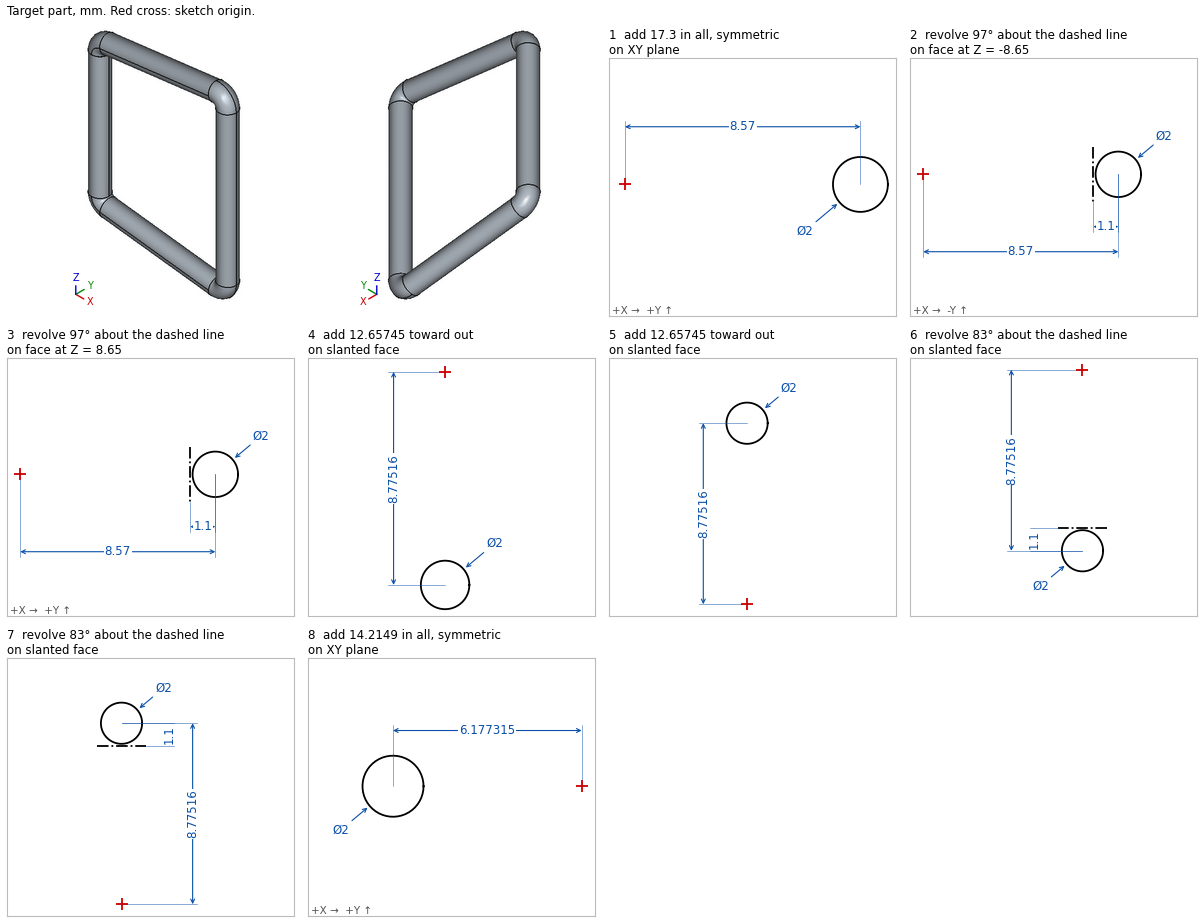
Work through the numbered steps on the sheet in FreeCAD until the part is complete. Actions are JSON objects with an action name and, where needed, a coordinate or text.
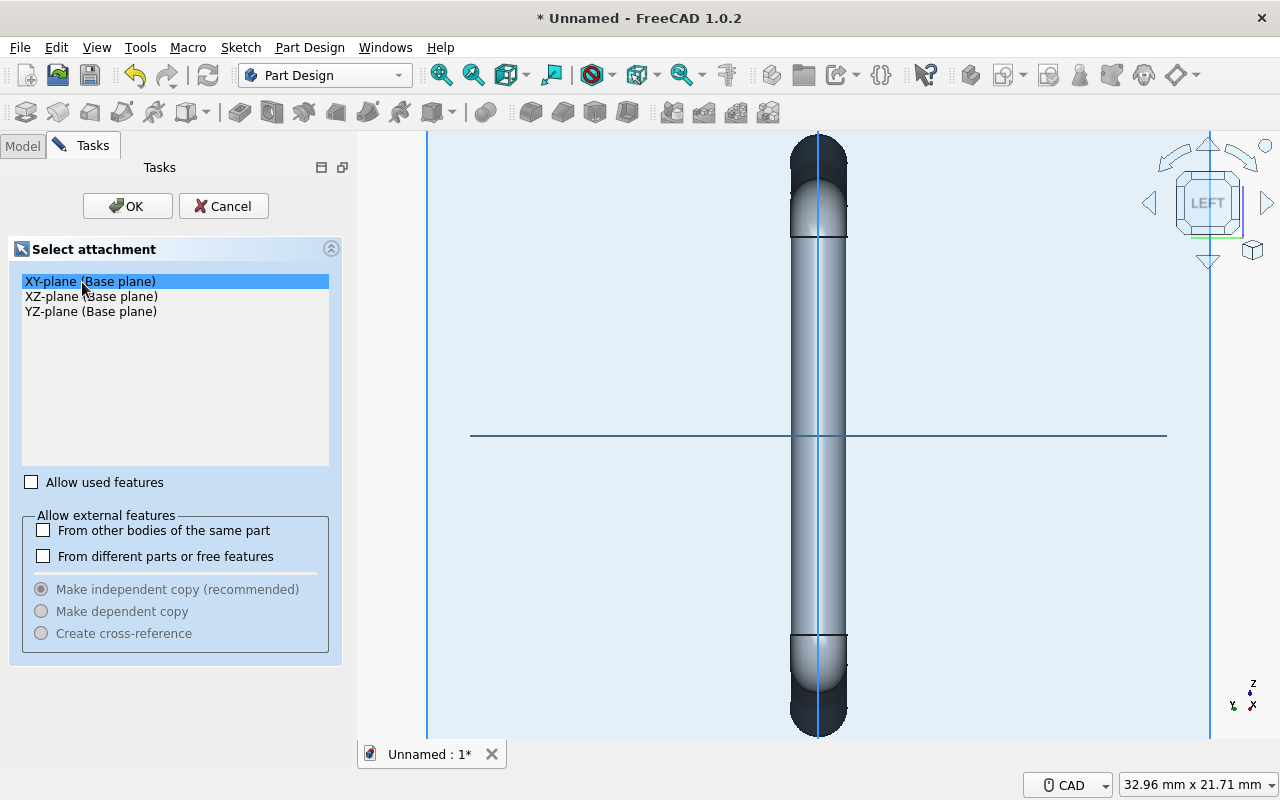
{"action": "left_click", "coordinate": [128, 206]}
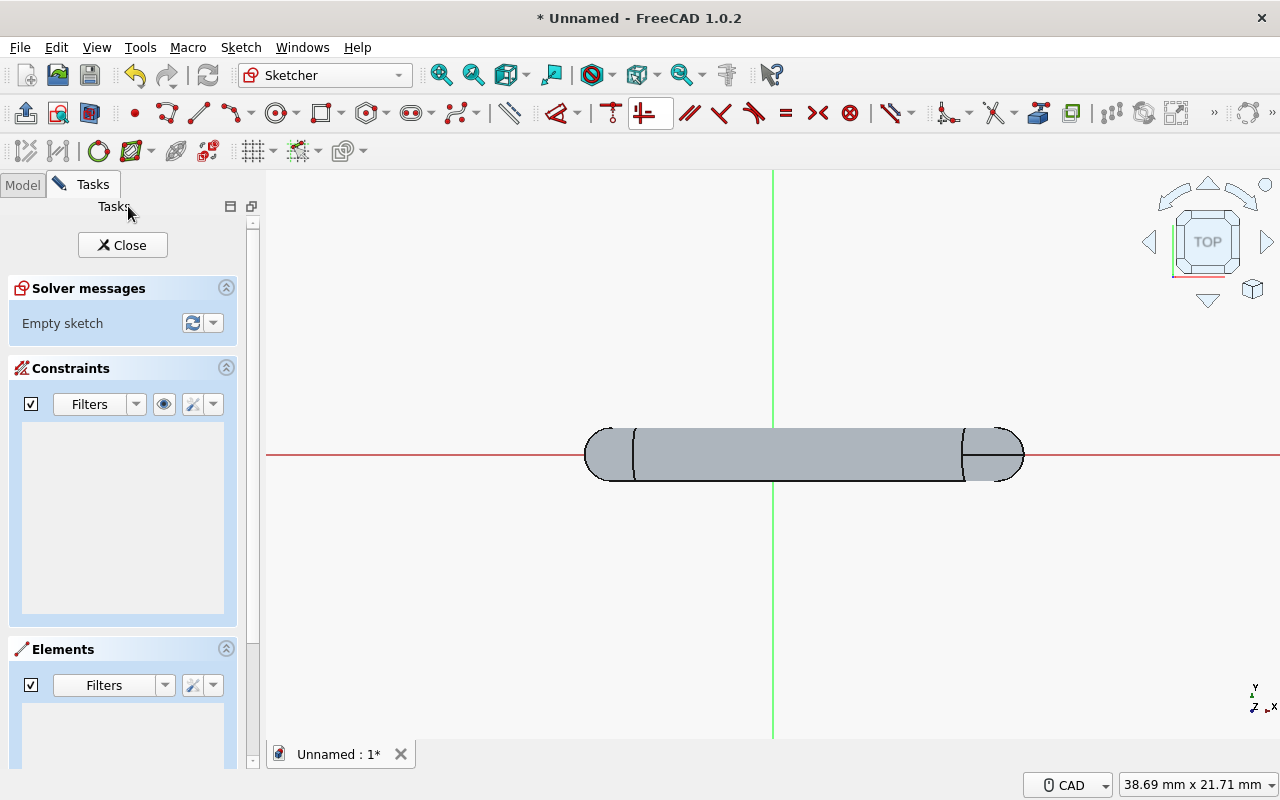
{"action": "left_click", "coordinate": [90, 114]}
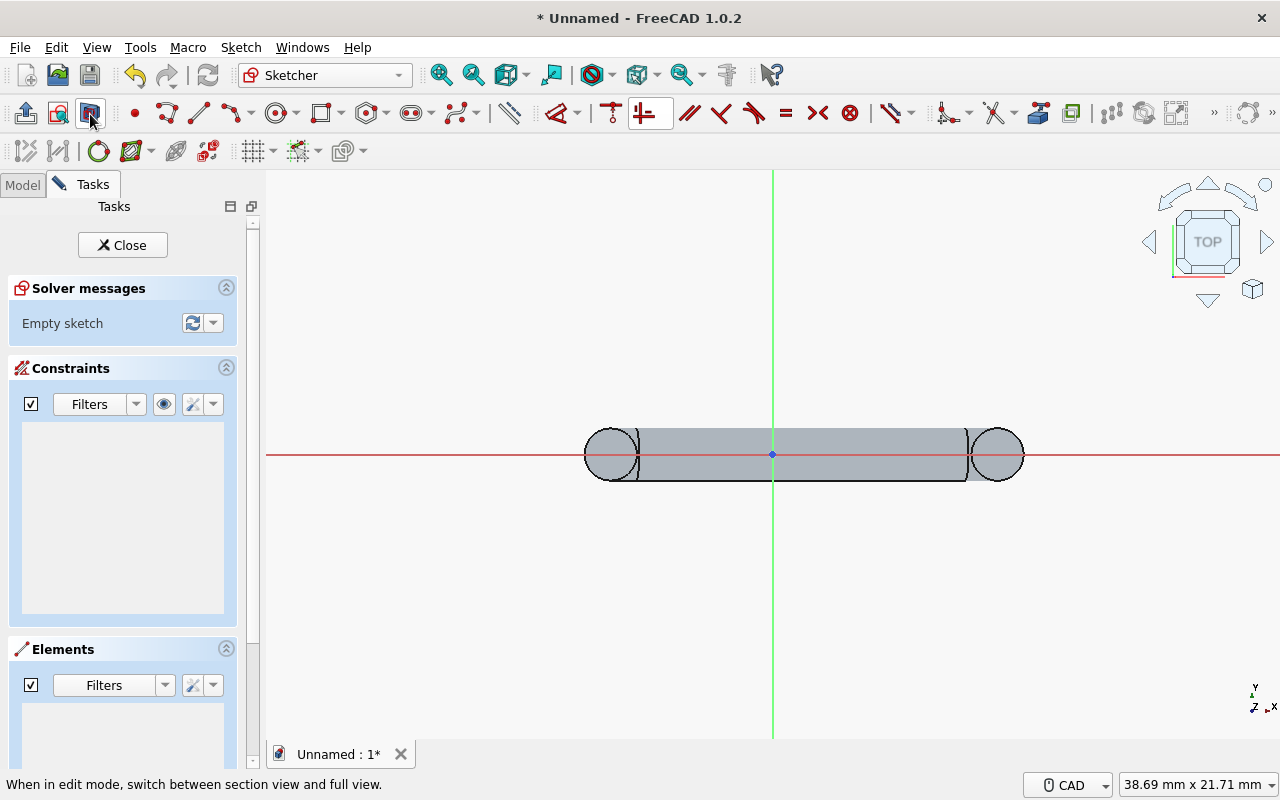
{"action": "scroll", "coordinate": [597, 454], "scroll_direction": "up", "scroll_amount": 10}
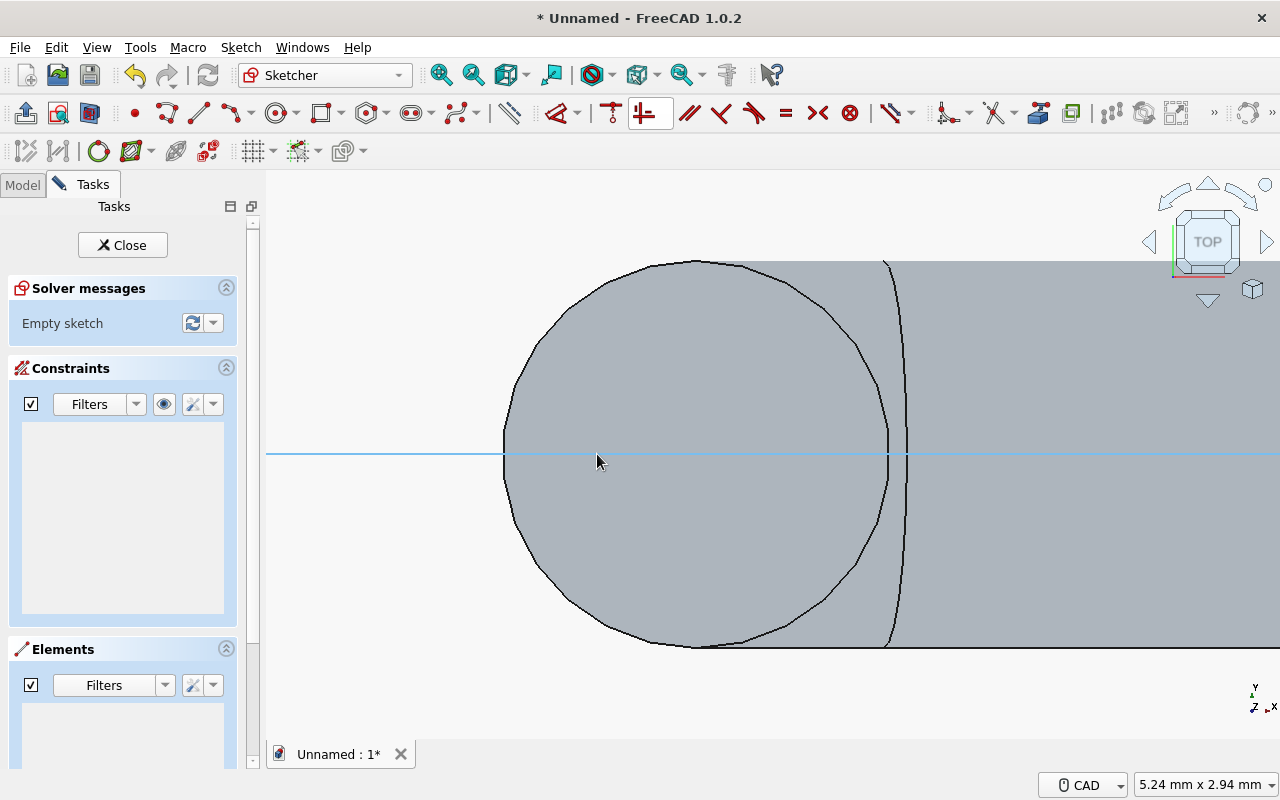
{"action": "left_click", "coordinate": [276, 114]}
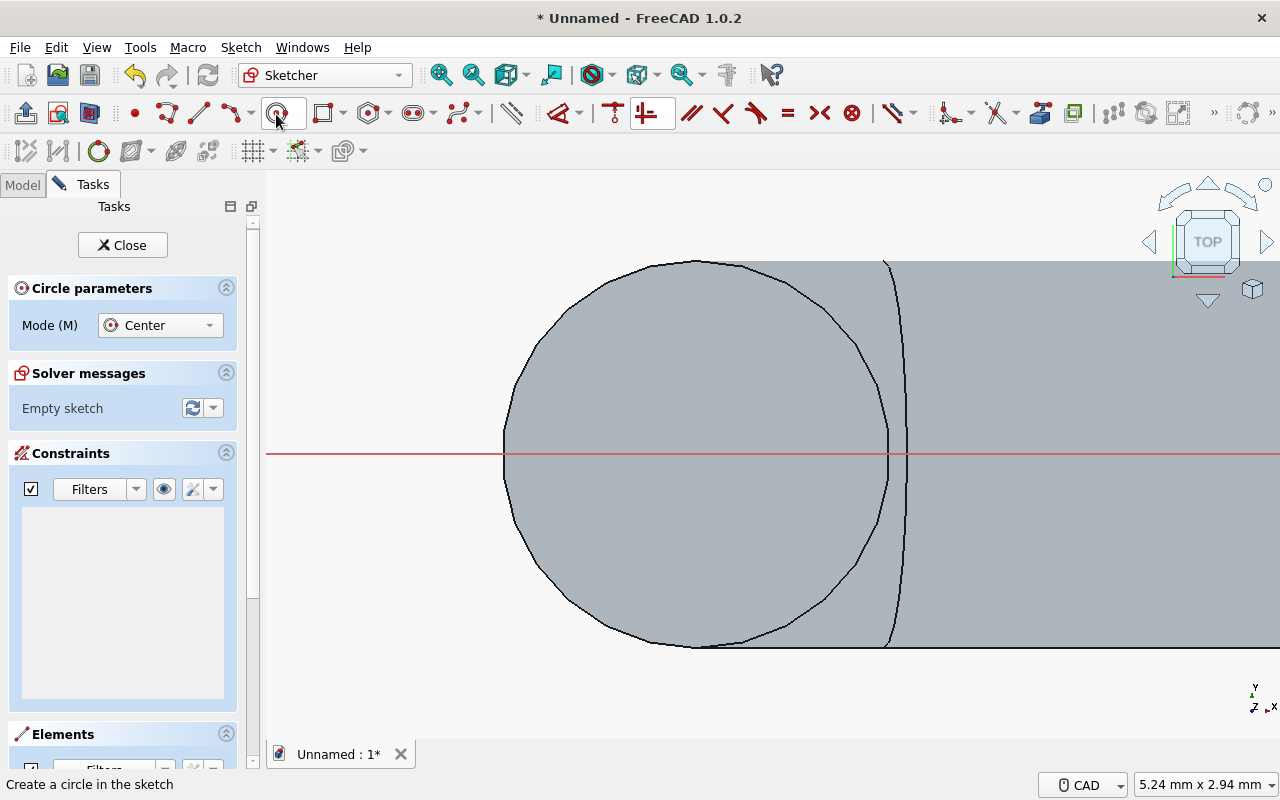
{"action": "left_click", "coordinate": [699, 454]}
{"action": "mouse_move", "coordinate": [836, 318]}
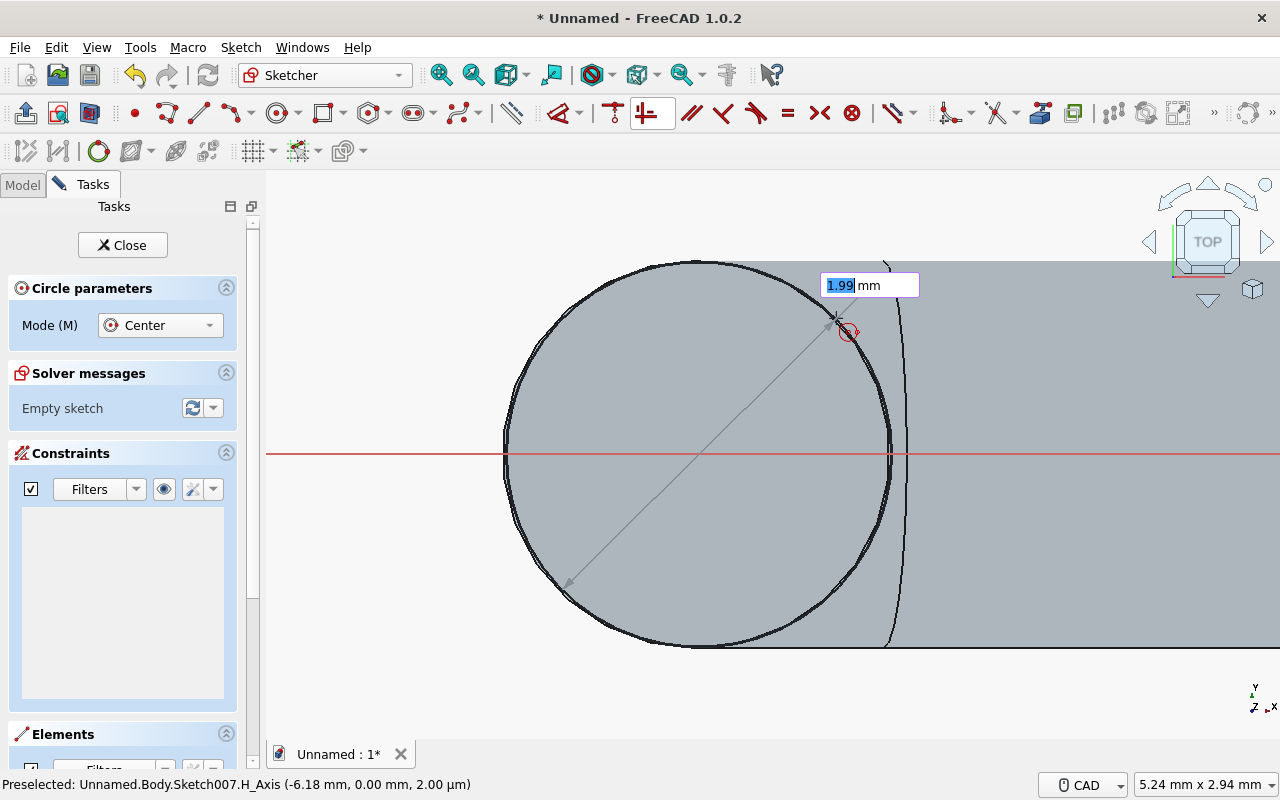
{"action": "type", "text": "2"}
{"action": "key", "text": "Return"}
{"action": "key", "text": "Escape"}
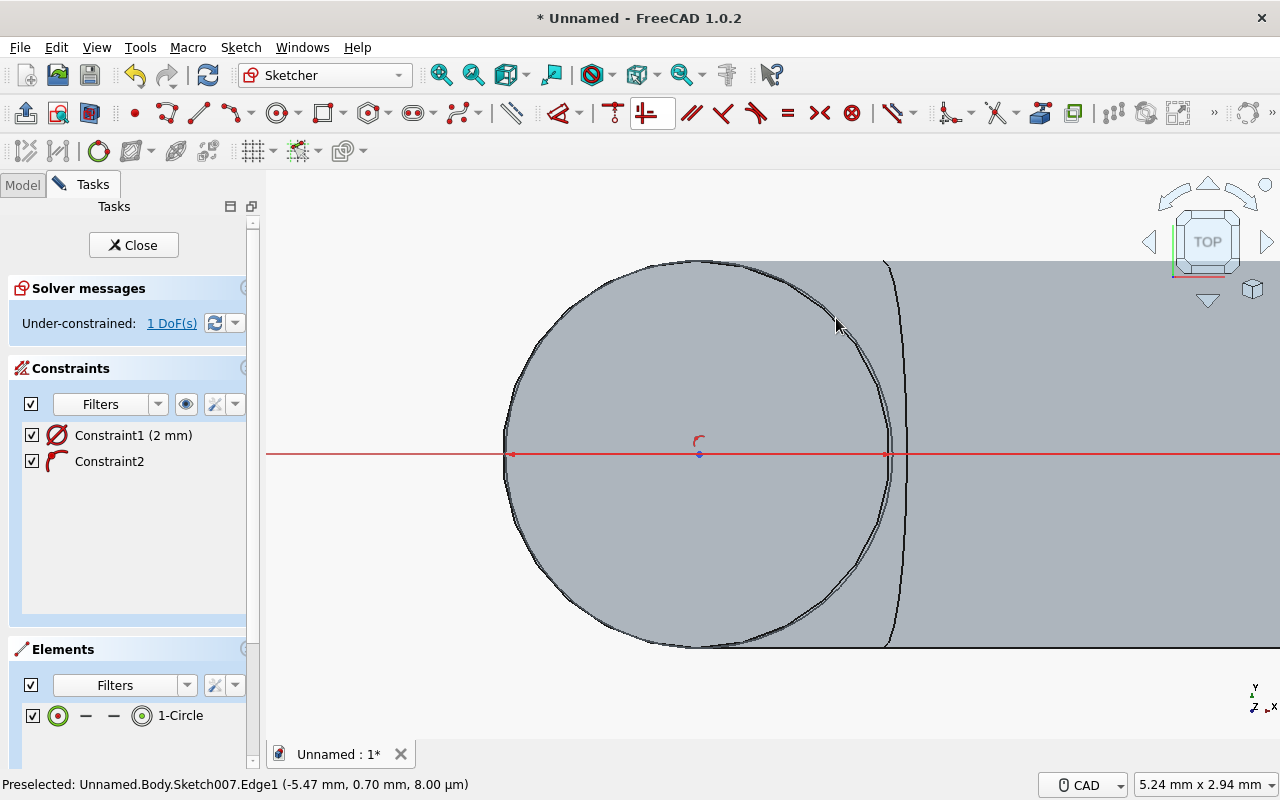
{"action": "left_click", "coordinate": [558, 114]}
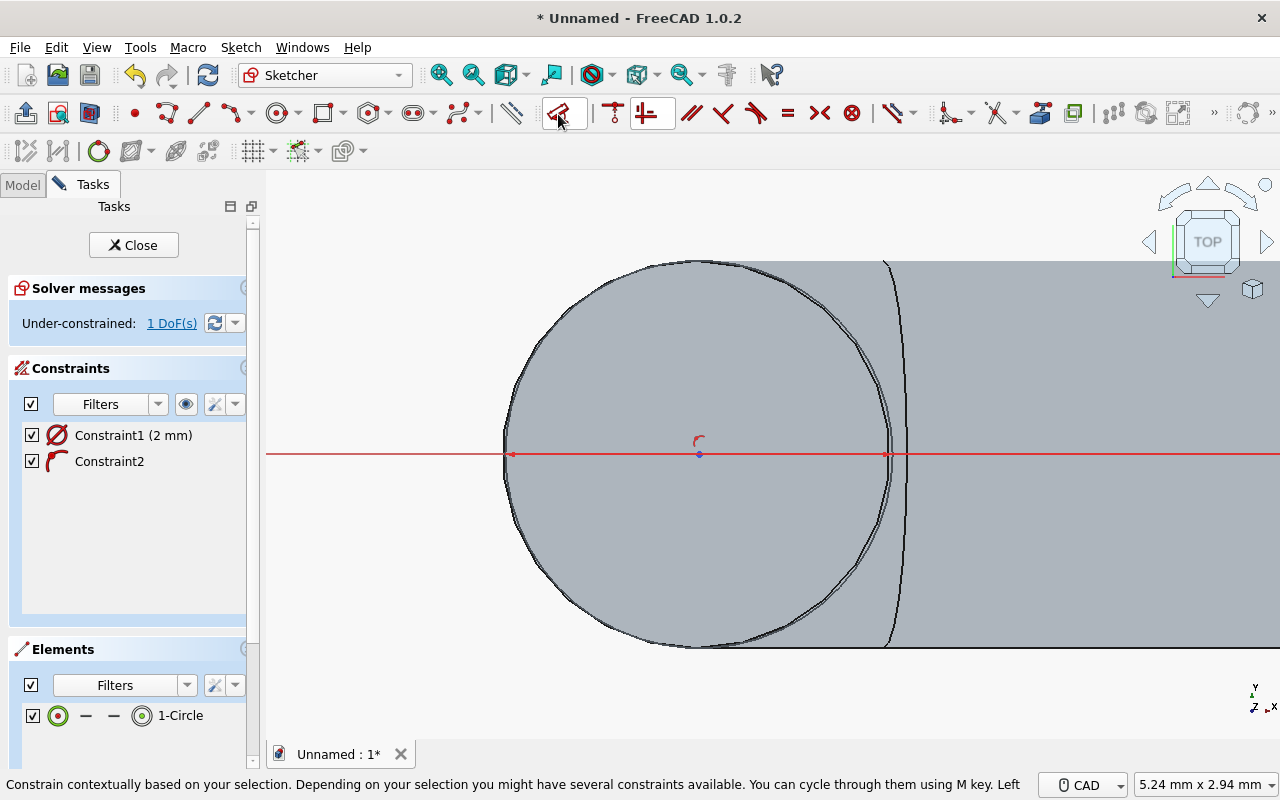
{"action": "left_click", "coordinate": [699, 454]}
{"action": "left_click", "coordinate": [907, 488]}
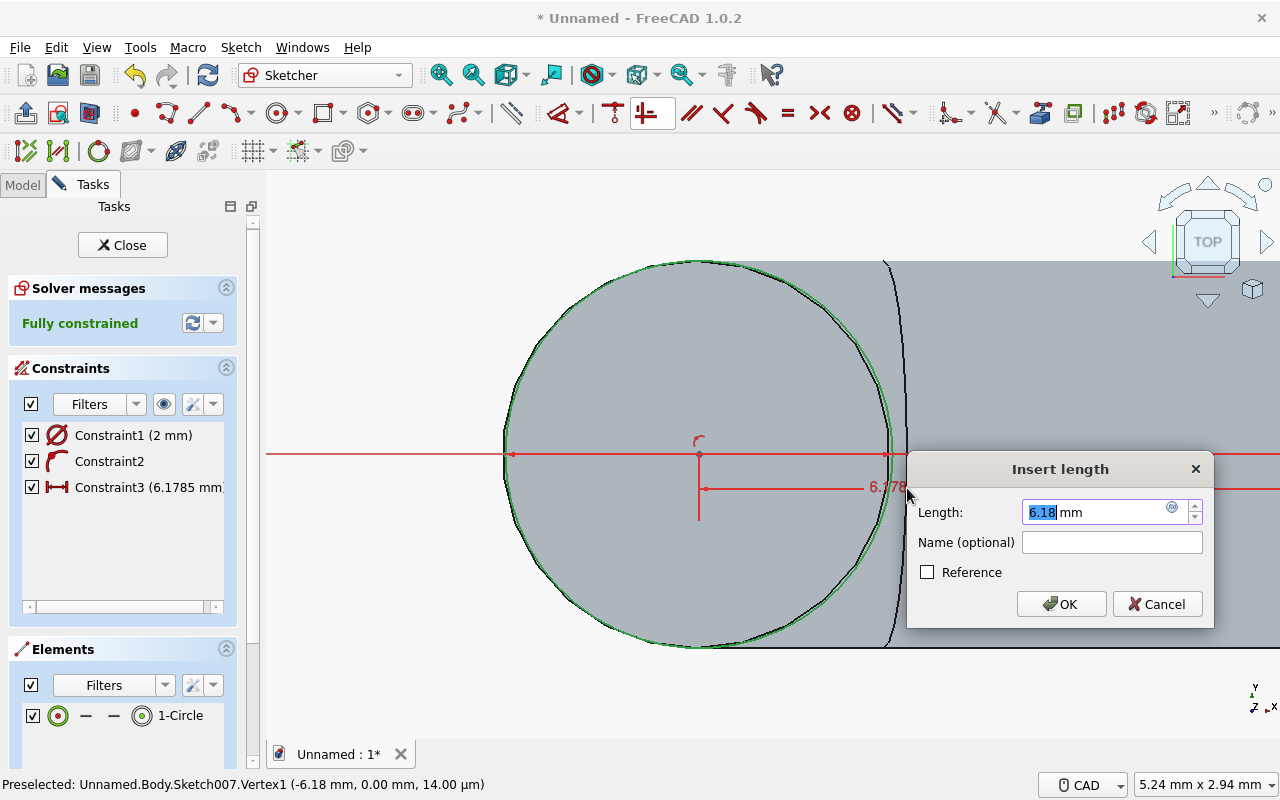
{"action": "type", "text": "6.177315"}
{"action": "key", "text": "Return"}
{"action": "key", "text": "Escape"}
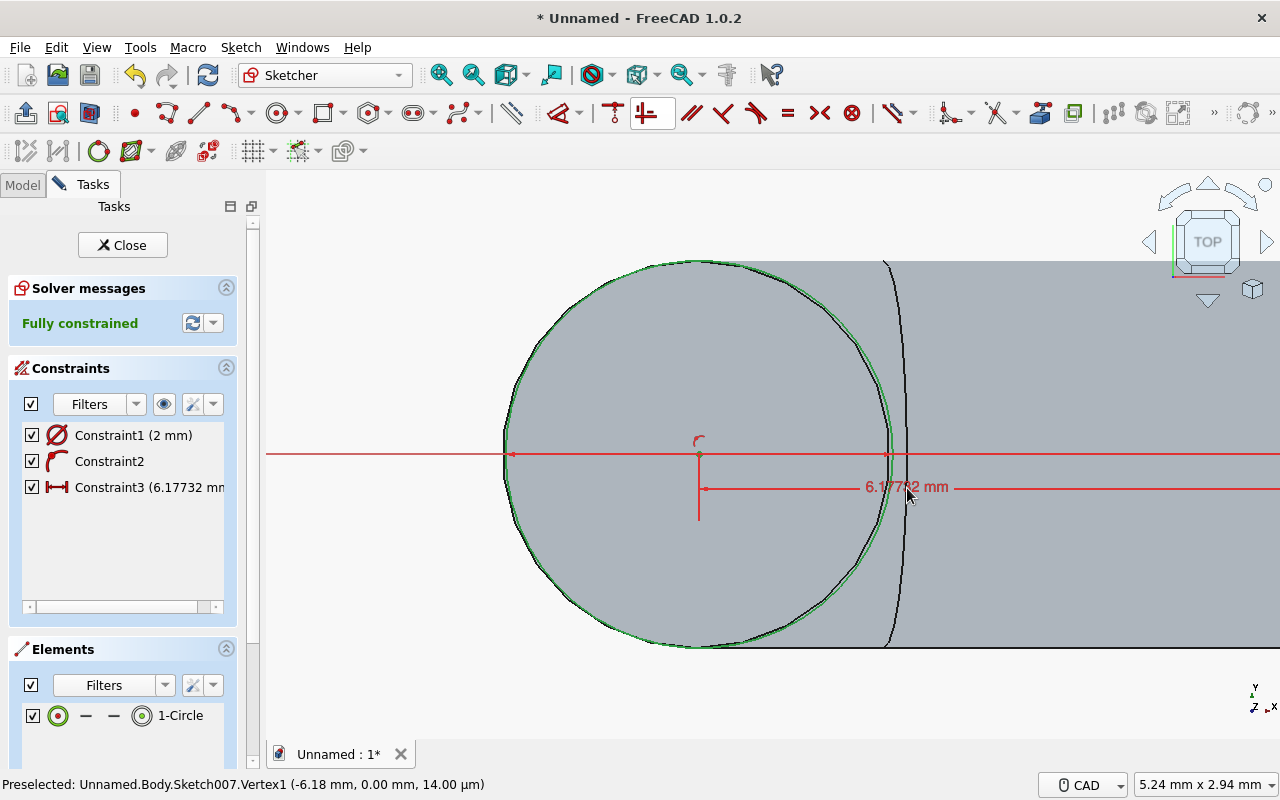
{"action": "left_click", "coordinate": [123, 245]}